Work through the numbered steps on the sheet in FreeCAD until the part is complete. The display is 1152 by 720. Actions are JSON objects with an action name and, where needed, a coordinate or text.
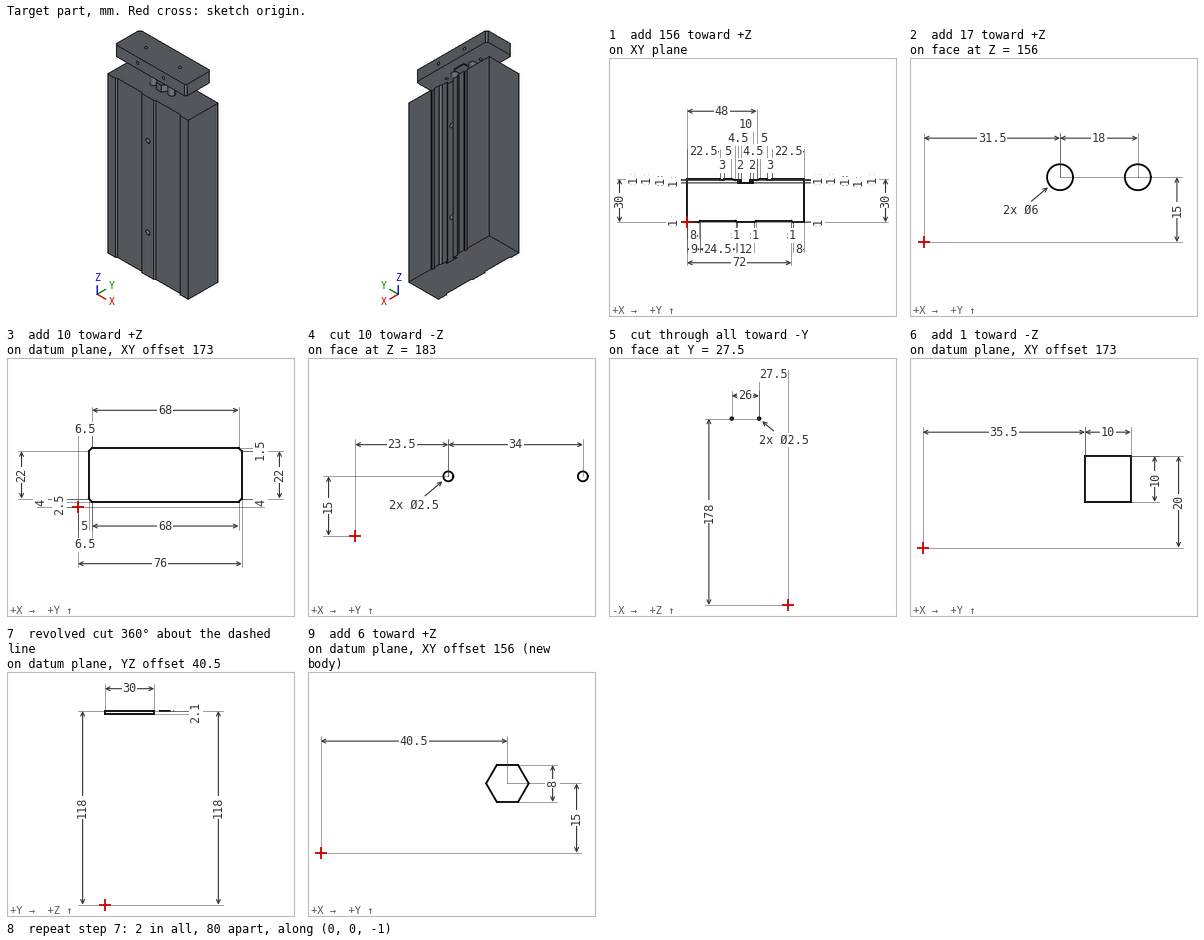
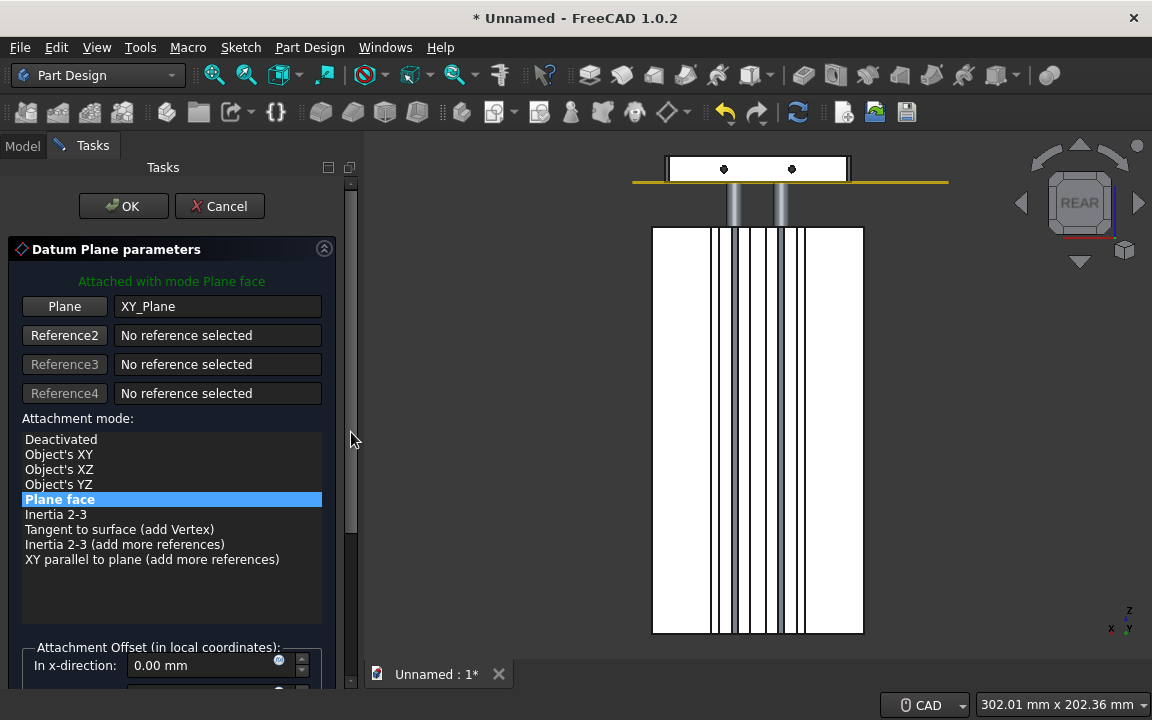
{"action": "left_click", "coordinate": [124, 206]}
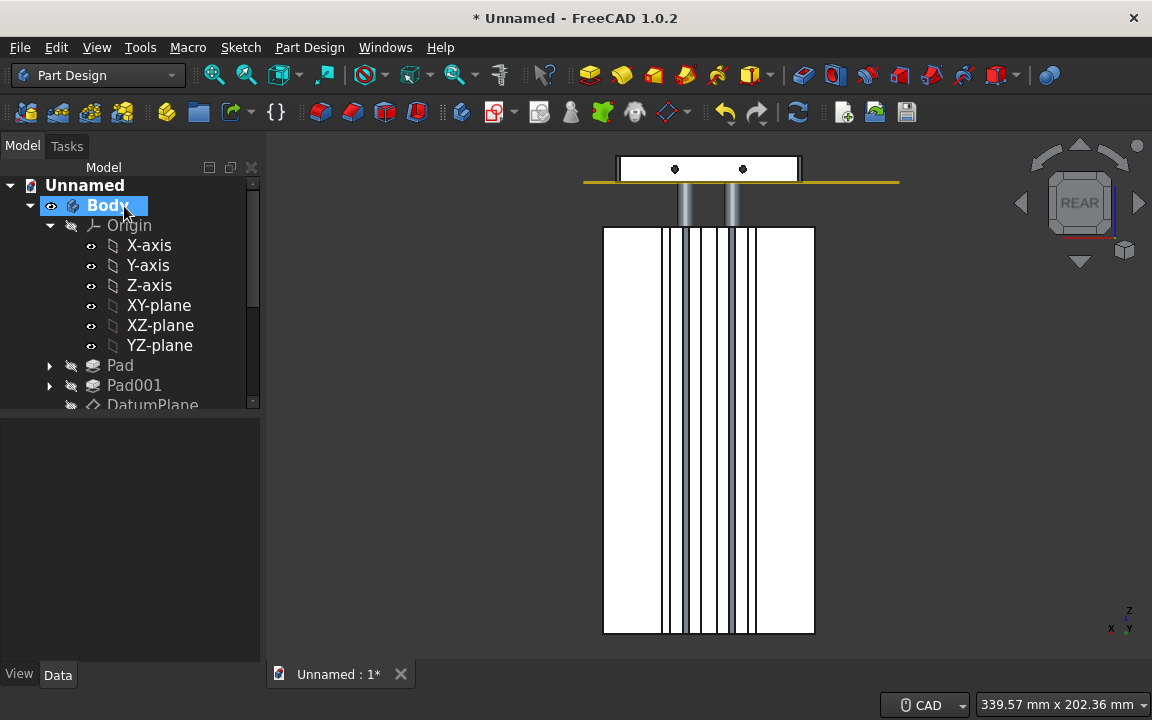
{"action": "scroll", "coordinate": [100, 301], "scroll_direction": "down", "scroll_amount": 3}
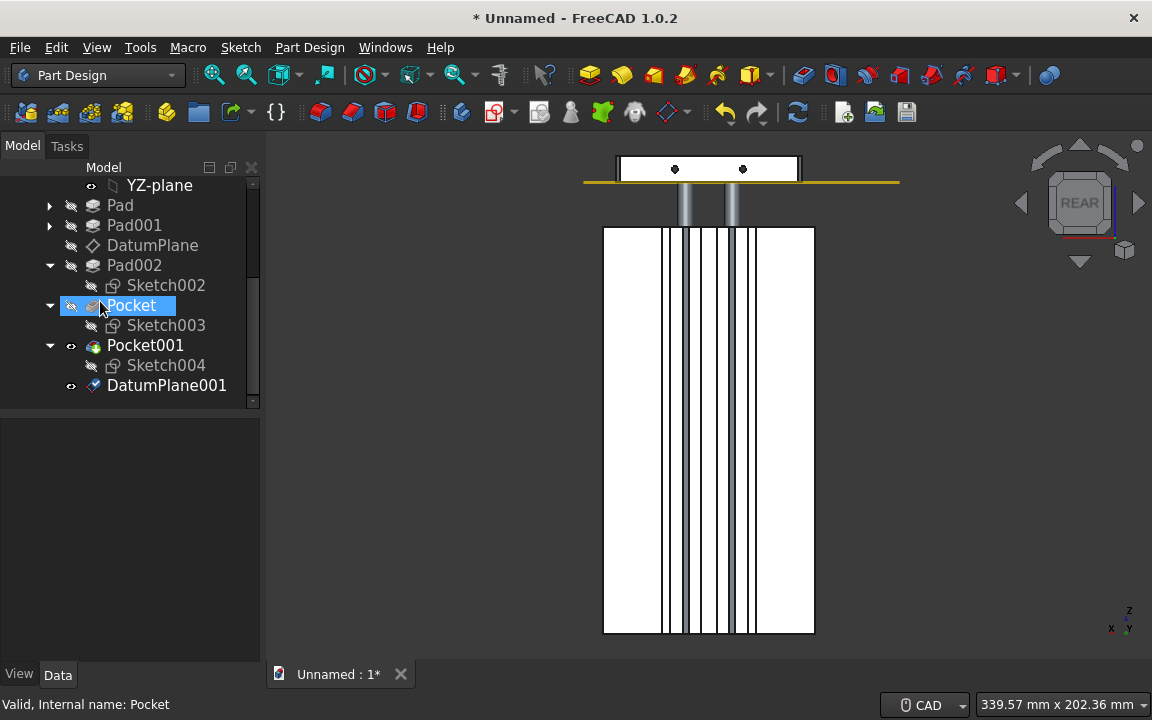
{"action": "left_click", "coordinate": [116, 386]}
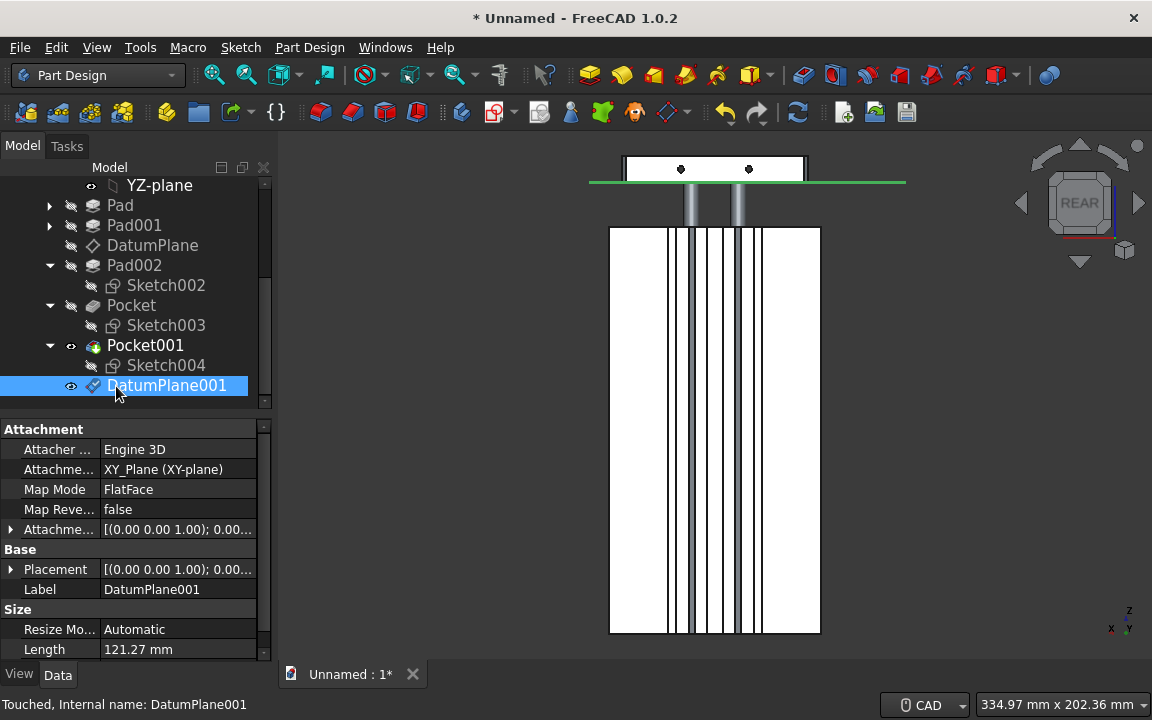
{"action": "left_click", "coordinate": [494, 112]}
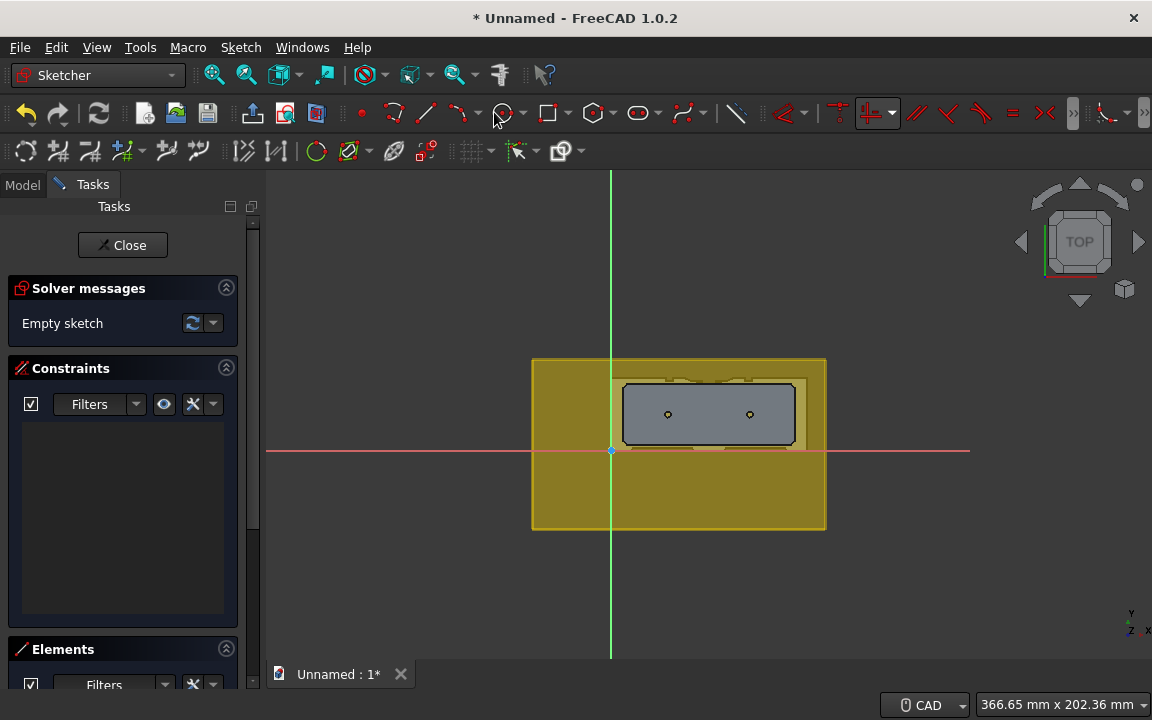
{"action": "key", "text": "q s"}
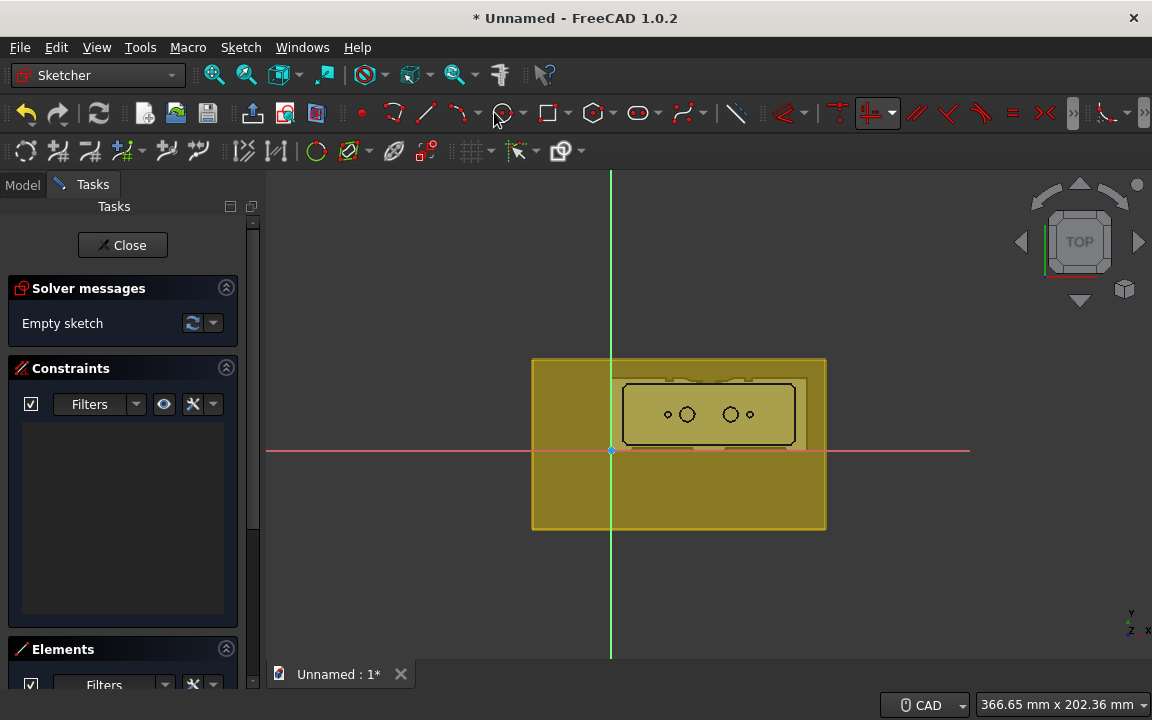
{"action": "scroll", "coordinate": [714, 414], "scroll_direction": "up", "scroll_amount": 13}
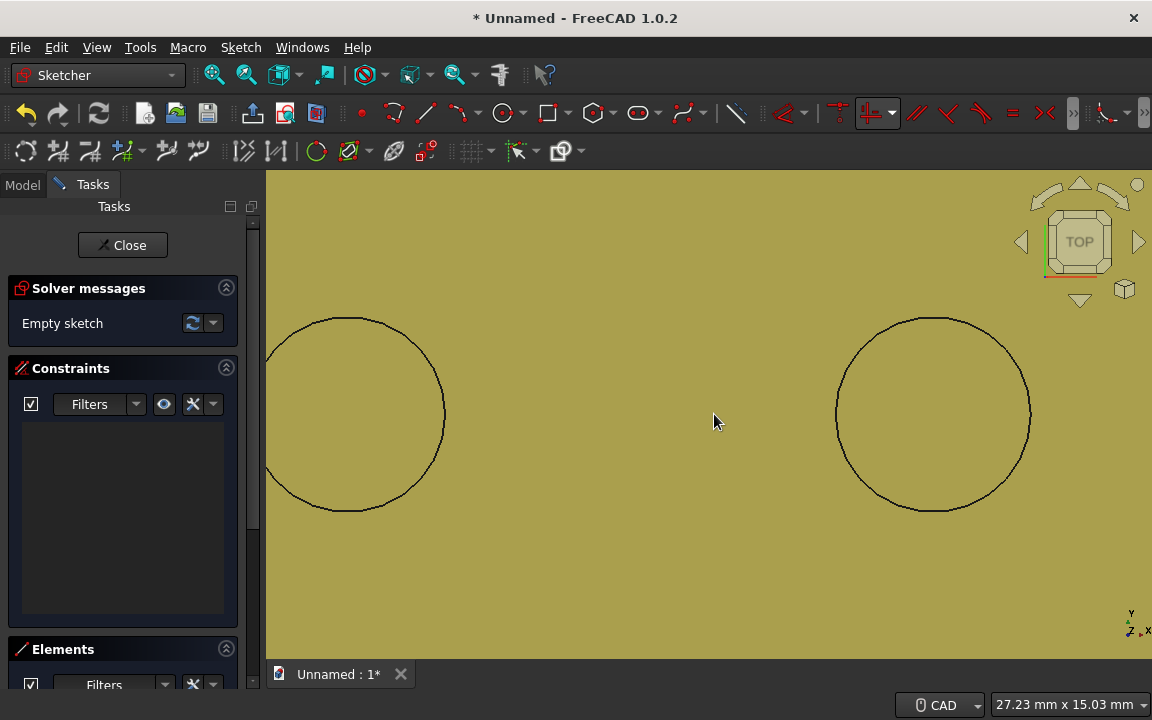
{"action": "key", "text": "g r"}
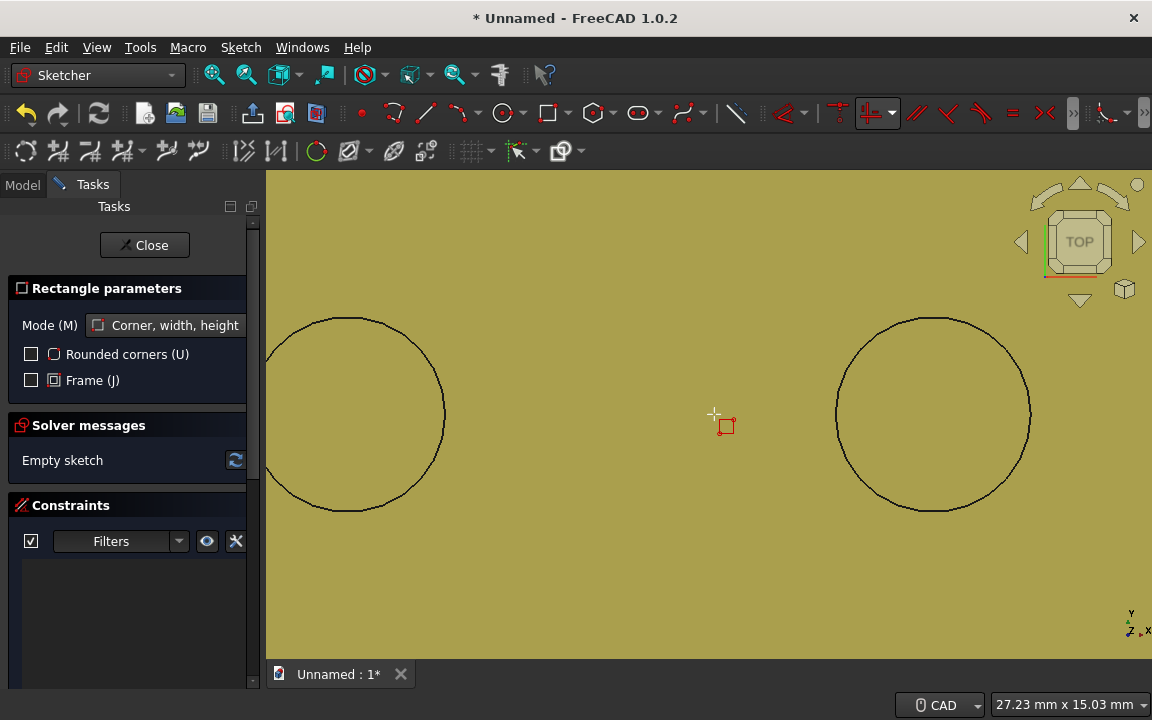
{"action": "left_click", "coordinate": [478, 252]}
{"action": "mouse_move", "coordinate": [803, 577]}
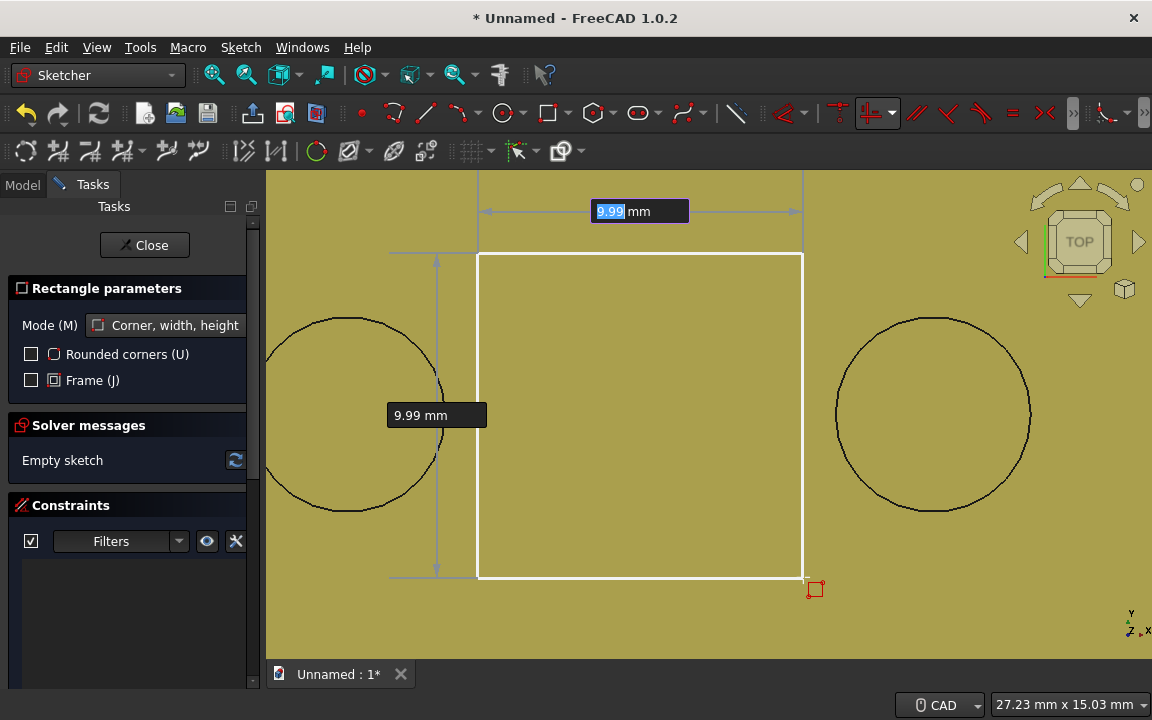
{"action": "type", "text": "10"}
{"action": "key", "text": "Tab"}
{"action": "type", "text": "10"}
{"action": "key", "text": "Return"}
{"action": "key", "text": "Escape"}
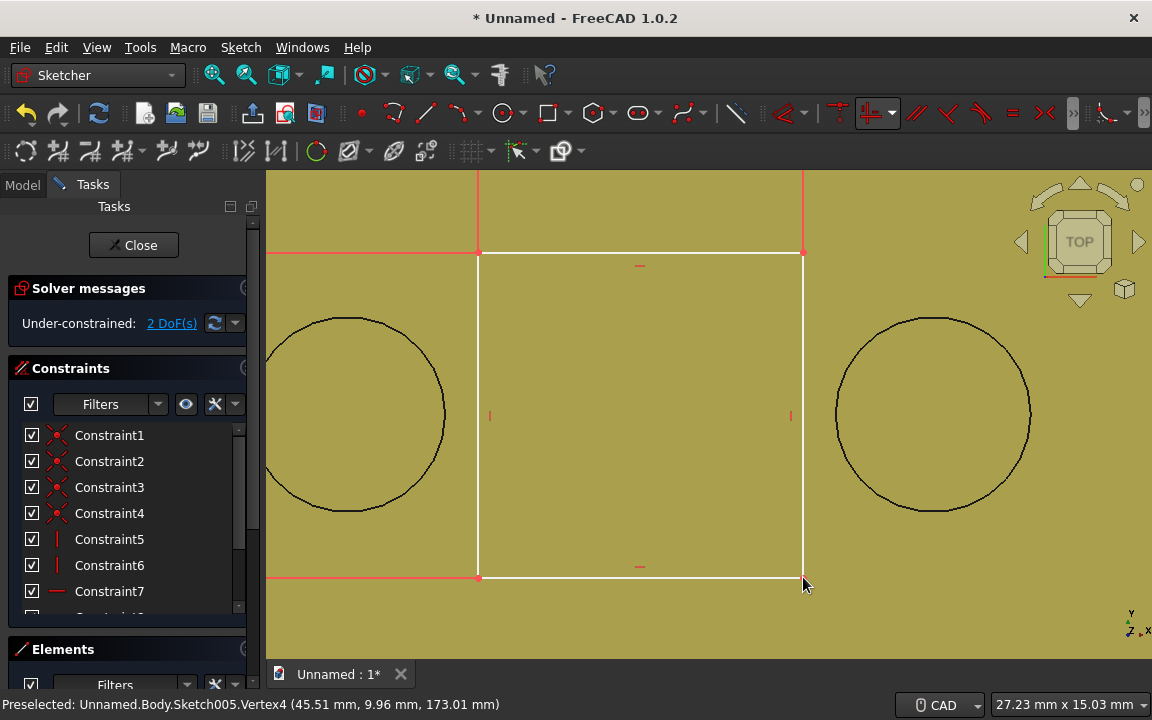
{"action": "key", "text": "d"}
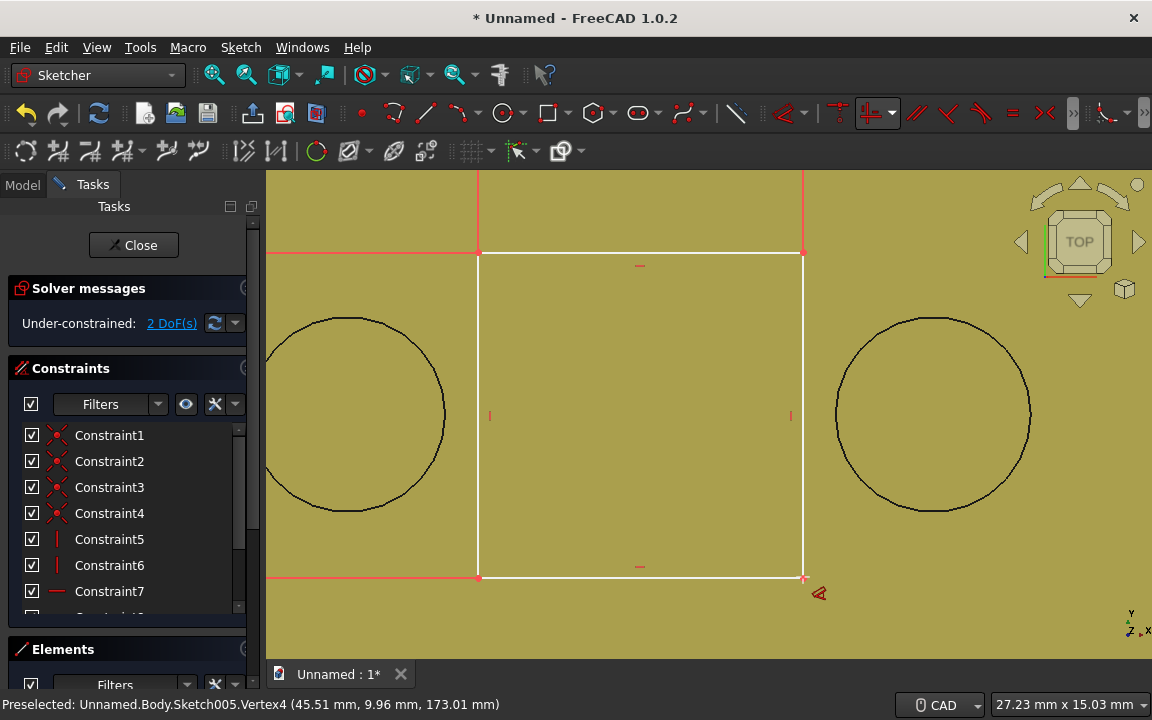
{"action": "left_click", "coordinate": [478, 253]}
{"action": "left_click", "coordinate": [512, 442]}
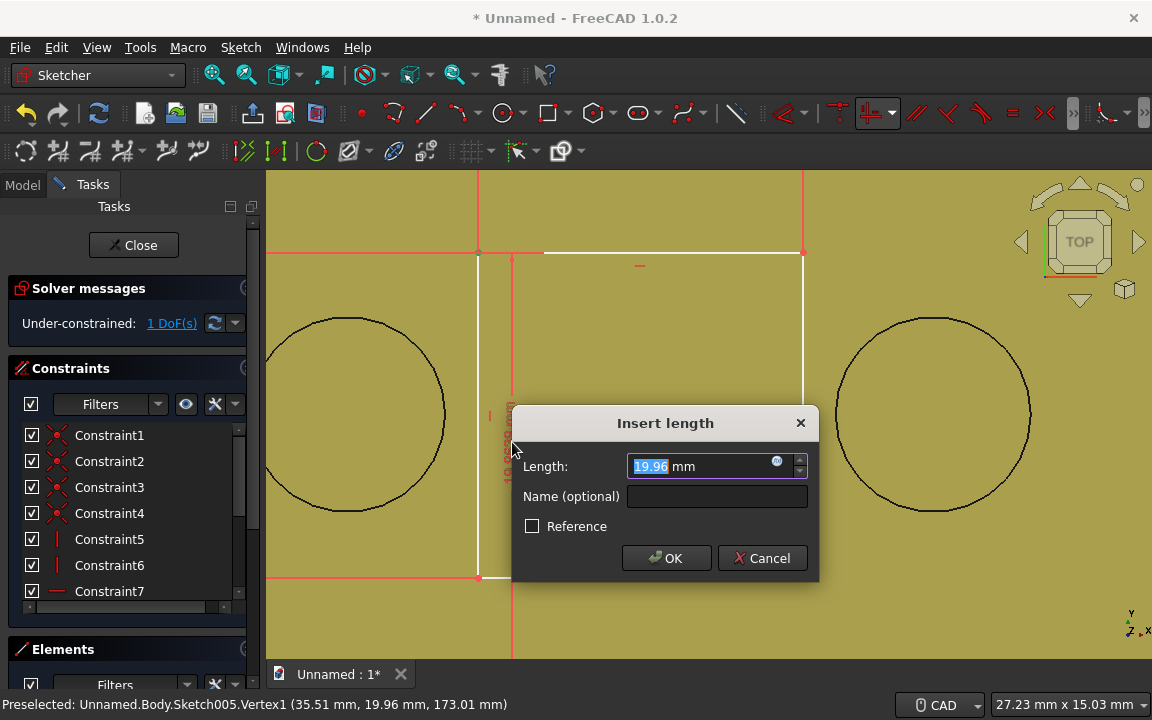
{"action": "type", "text": "20"}
{"action": "key", "text": "Return"}